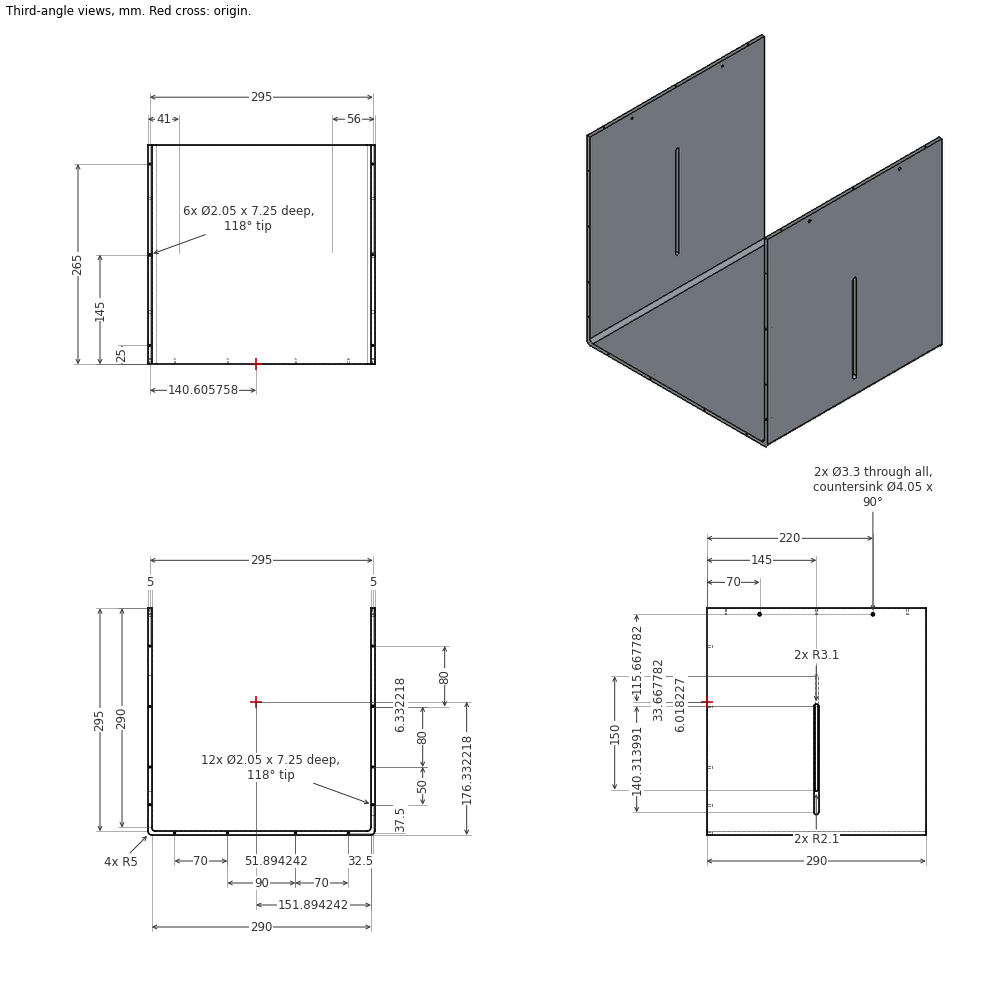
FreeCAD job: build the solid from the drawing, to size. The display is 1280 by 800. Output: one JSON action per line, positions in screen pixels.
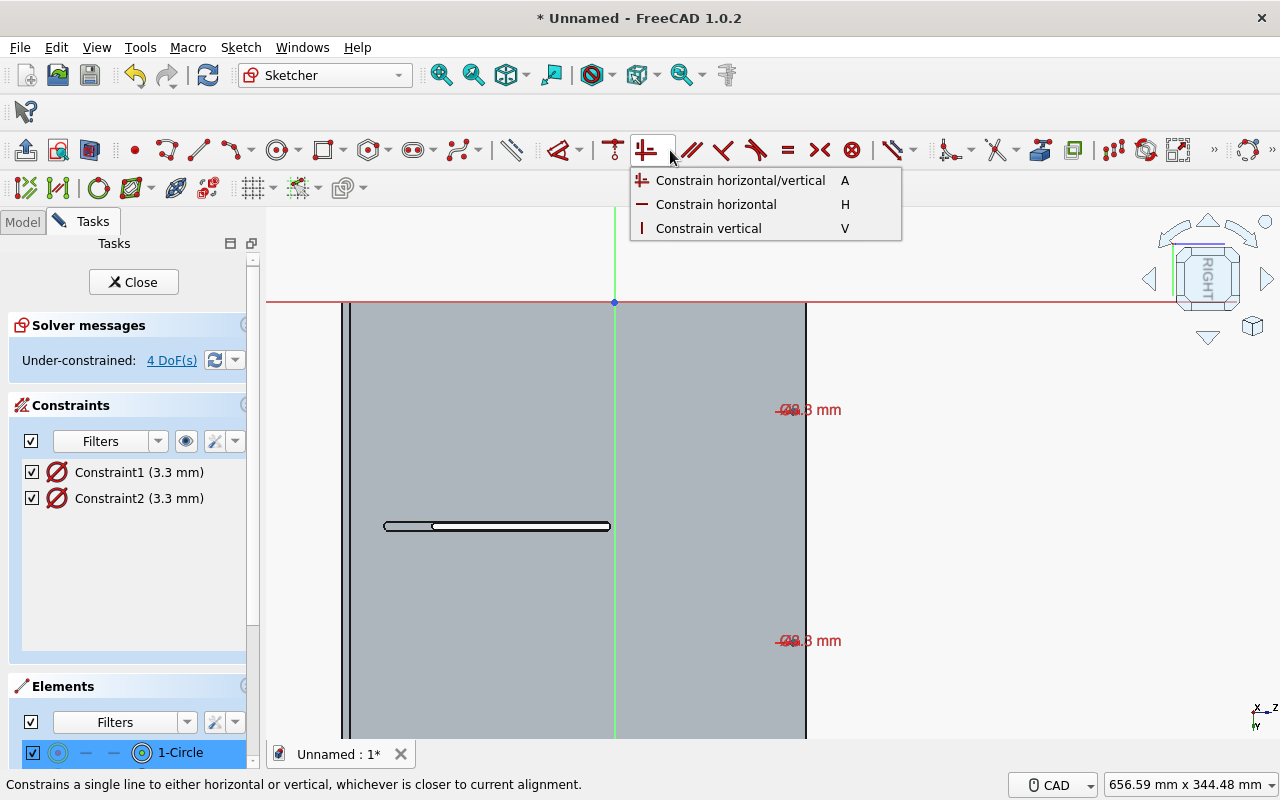
{"action": "left_click", "coordinate": [766, 228]}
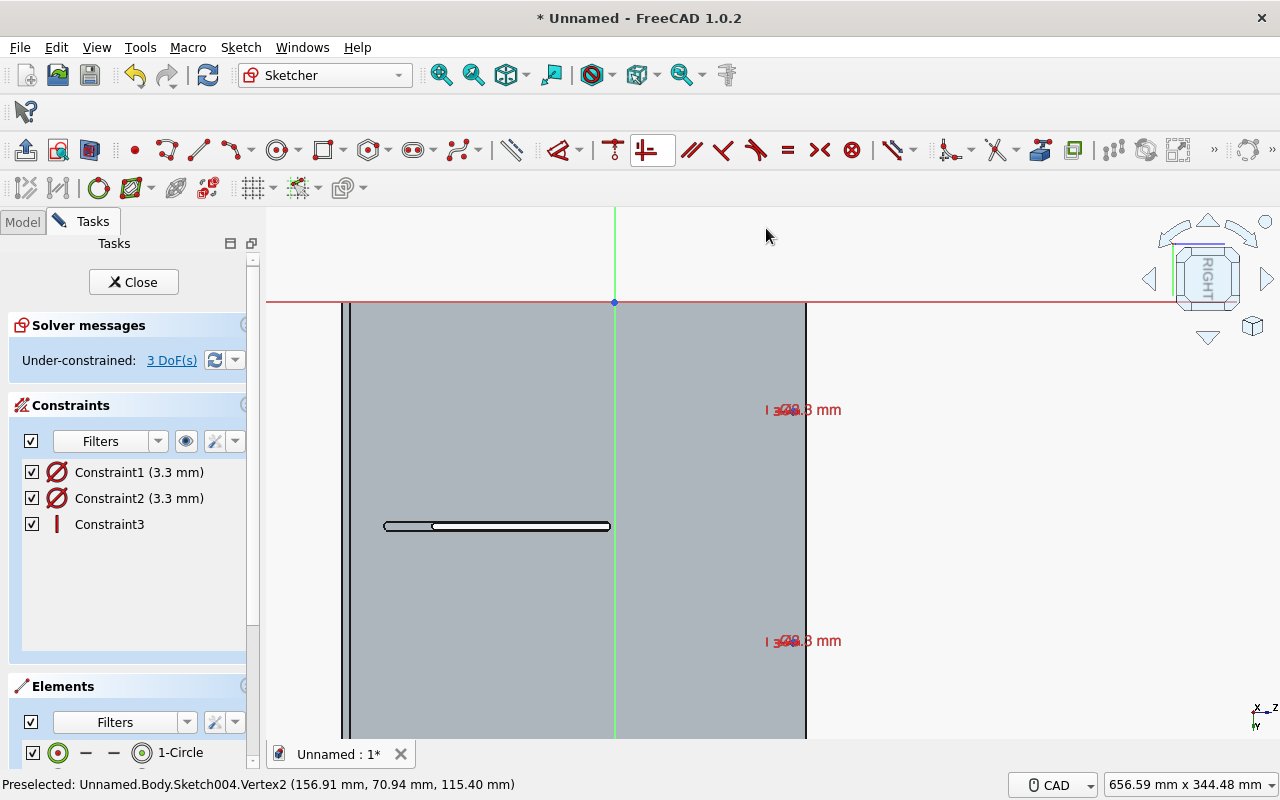
{"action": "left_click", "coordinate": [558, 150]}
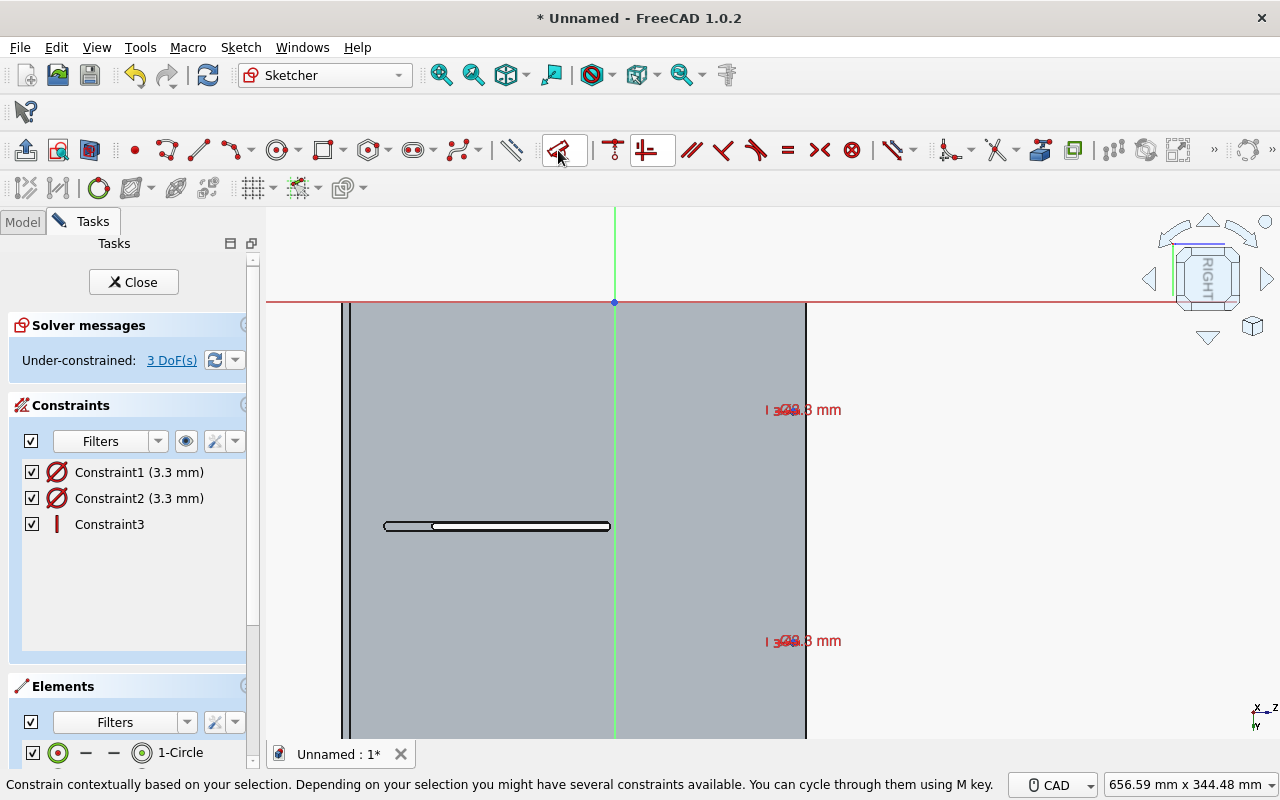
{"action": "left_click", "coordinate": [793, 412]}
{"action": "left_click", "coordinate": [581, 357]}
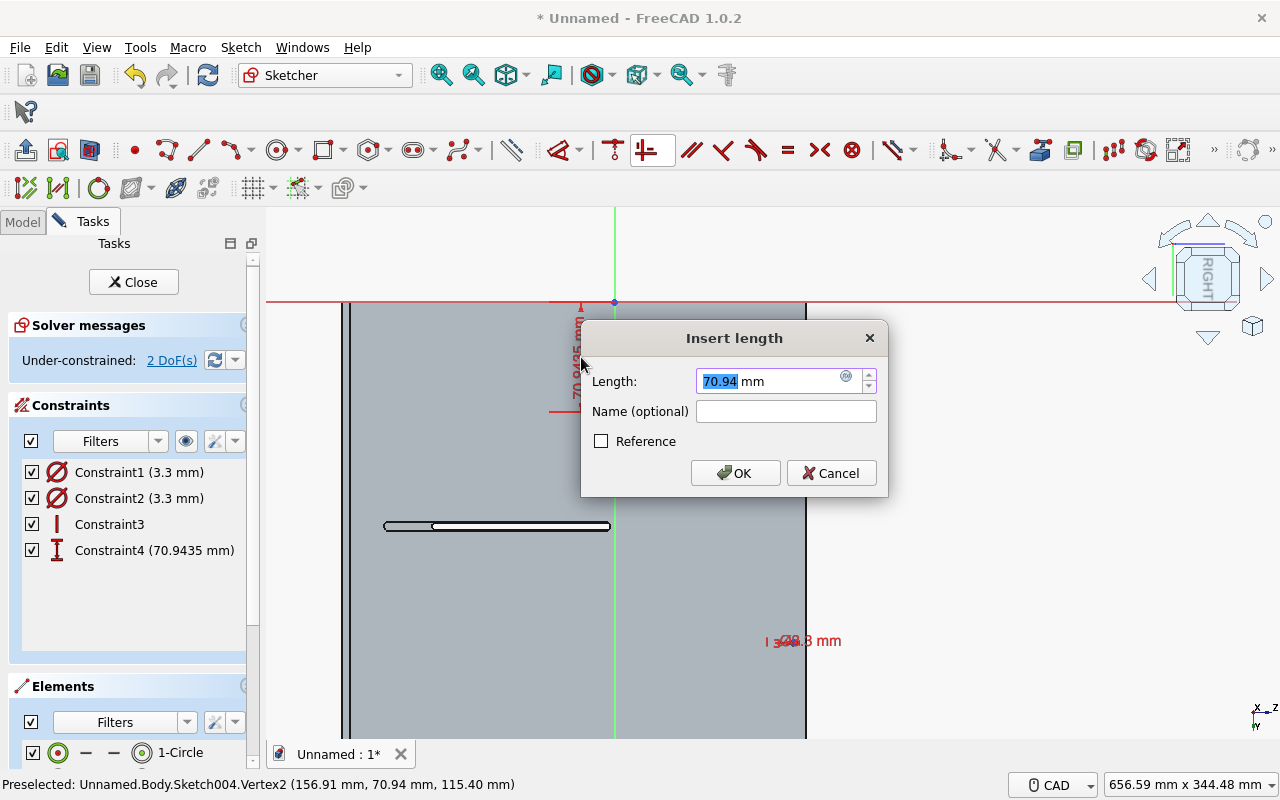
{"action": "type", "text": "70"}
{"action": "key", "text": "Return"}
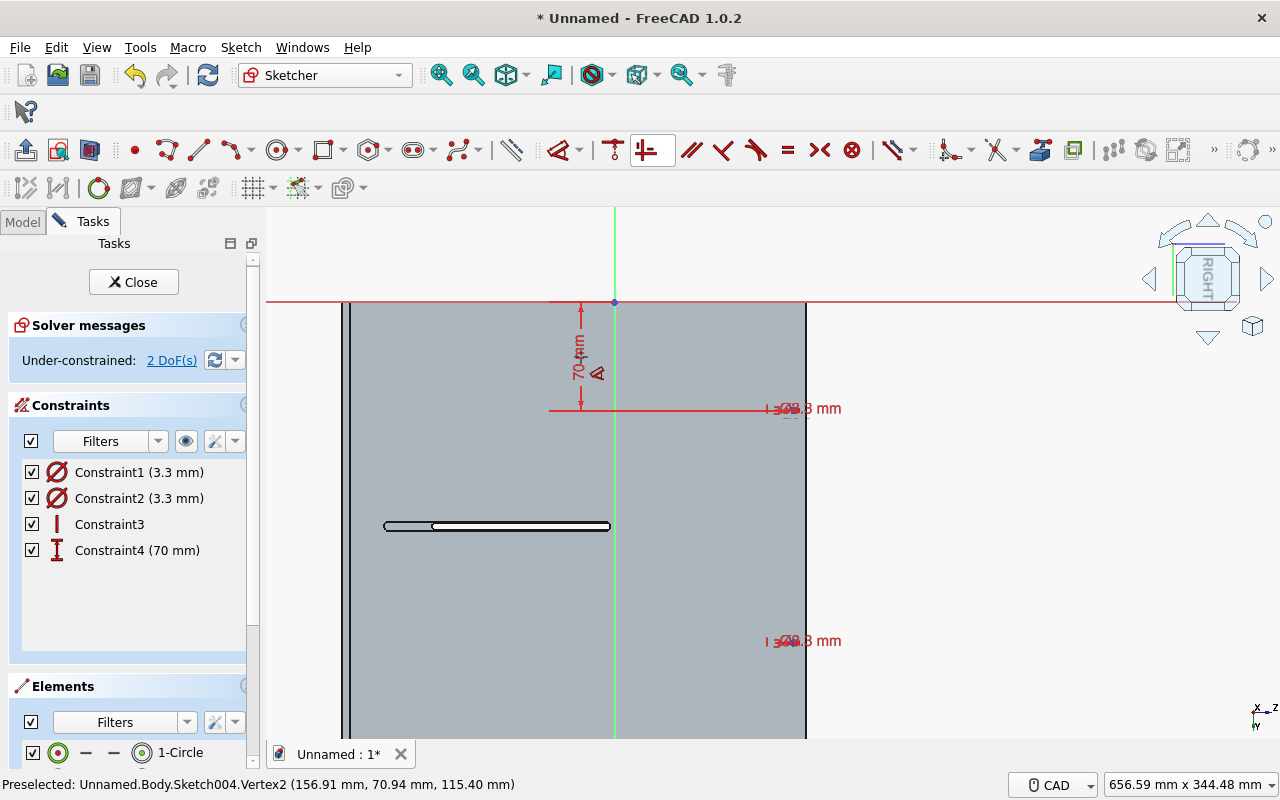
{"action": "left_click", "coordinate": [793, 643]}
{"action": "left_click", "coordinate": [581, 473]}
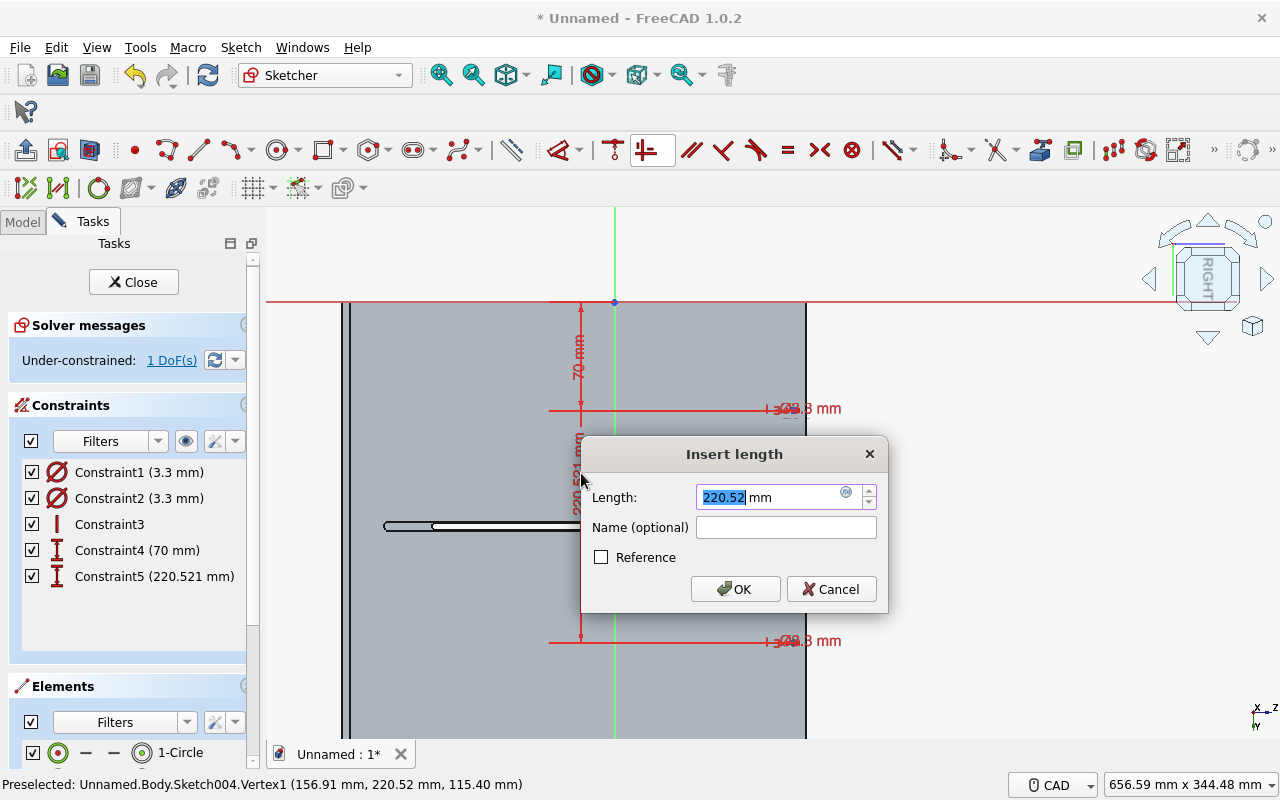
{"action": "type", "text": "220"}
{"action": "key", "text": "Return"}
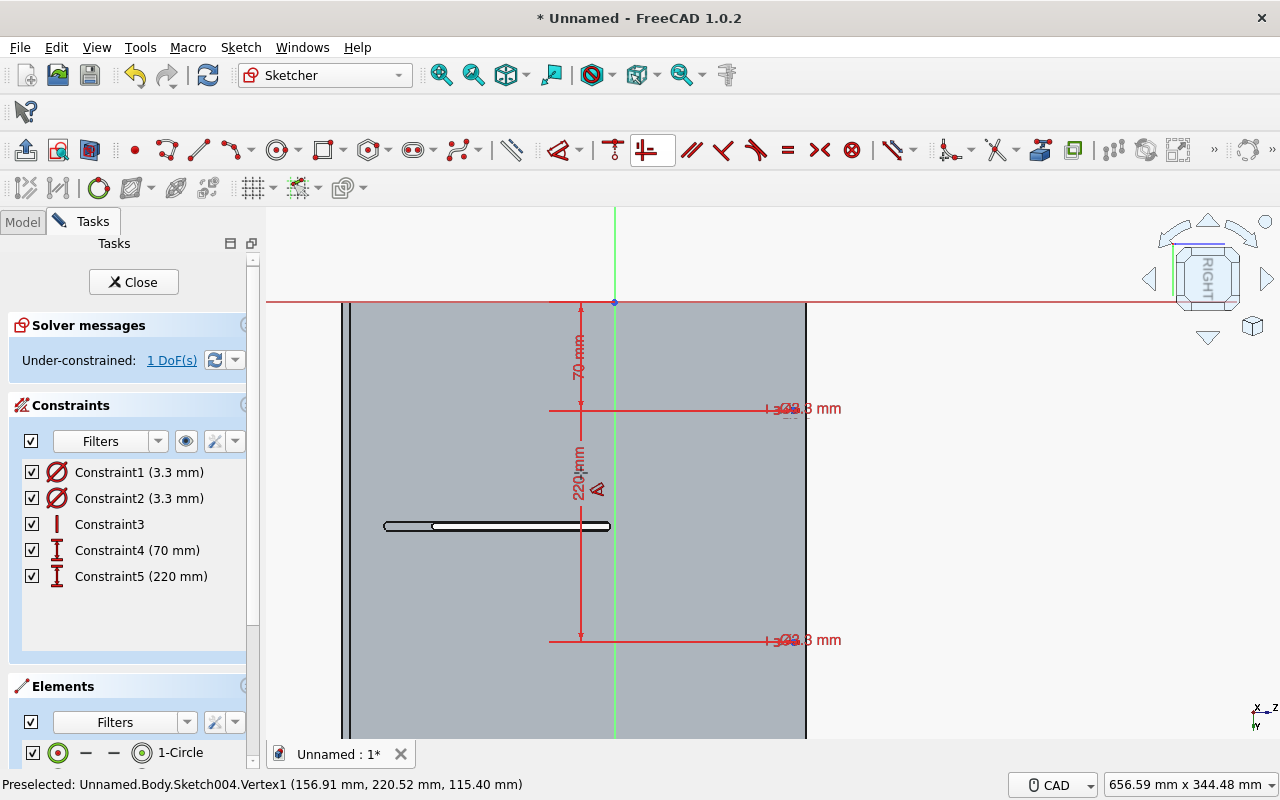
{"action": "left_click", "coordinate": [793, 642]}
{"action": "left_click", "coordinate": [704, 268]}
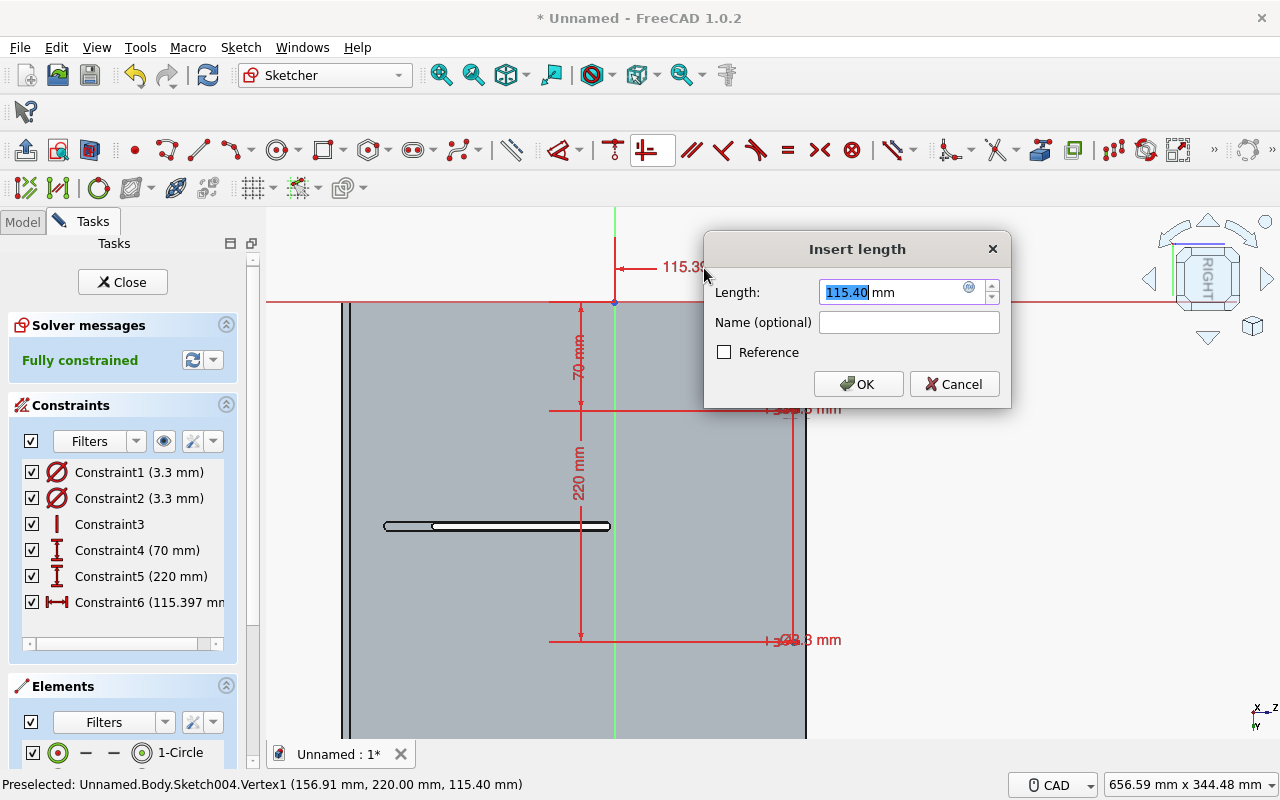
{"action": "type", "text": "115.667782"}
{"action": "key", "text": "Return"}
{"action": "key", "text": "Escape"}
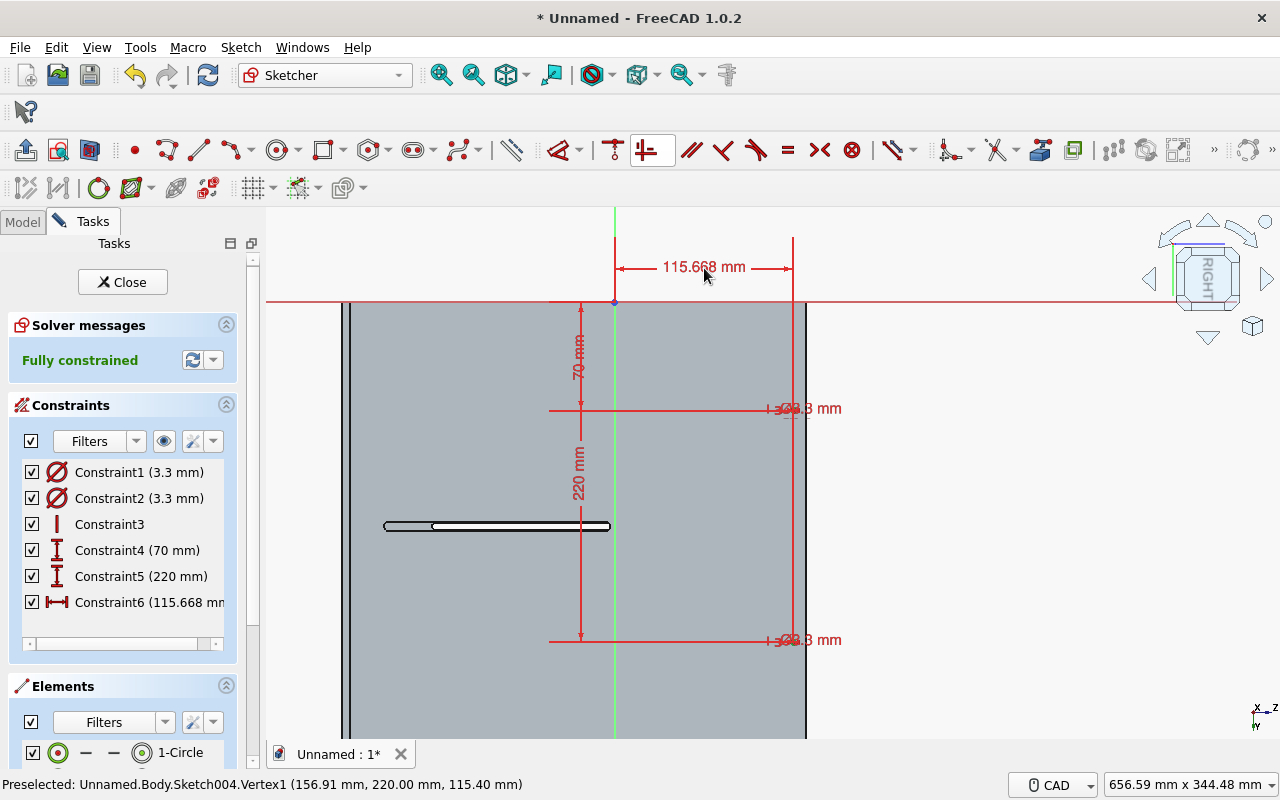
{"action": "left_click", "coordinate": [123, 282]}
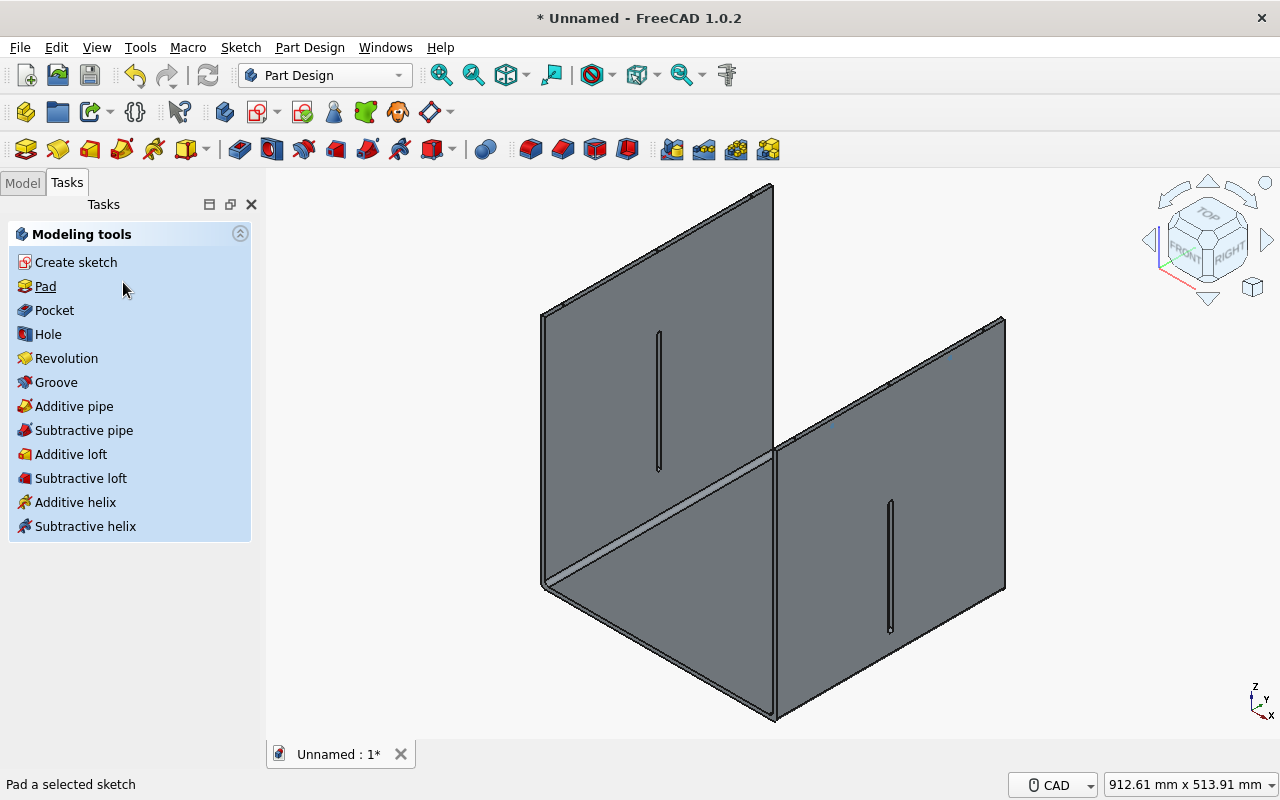
{"action": "left_click", "coordinate": [272, 150]}